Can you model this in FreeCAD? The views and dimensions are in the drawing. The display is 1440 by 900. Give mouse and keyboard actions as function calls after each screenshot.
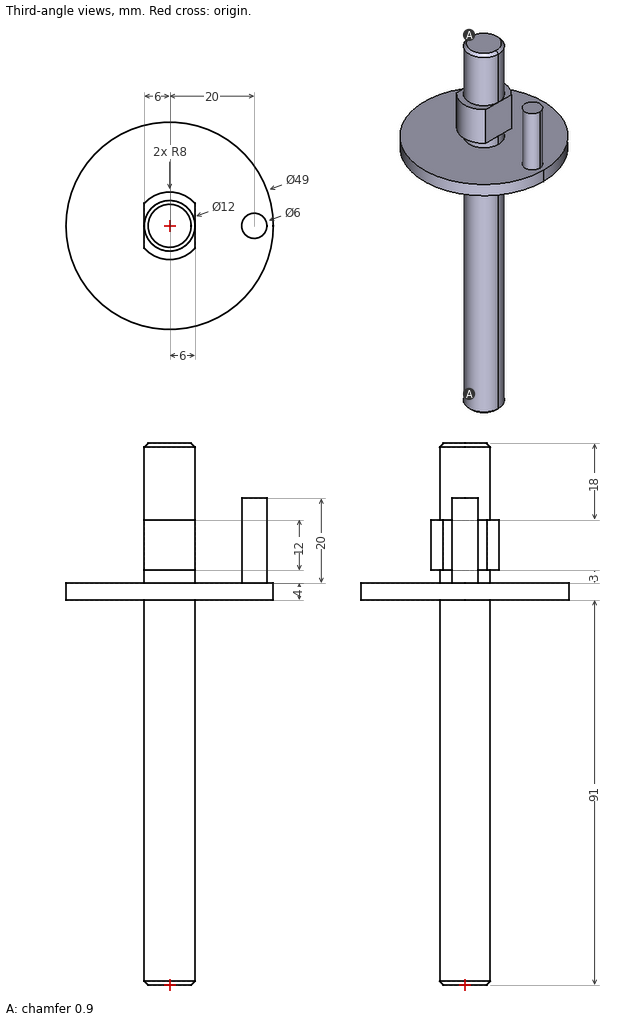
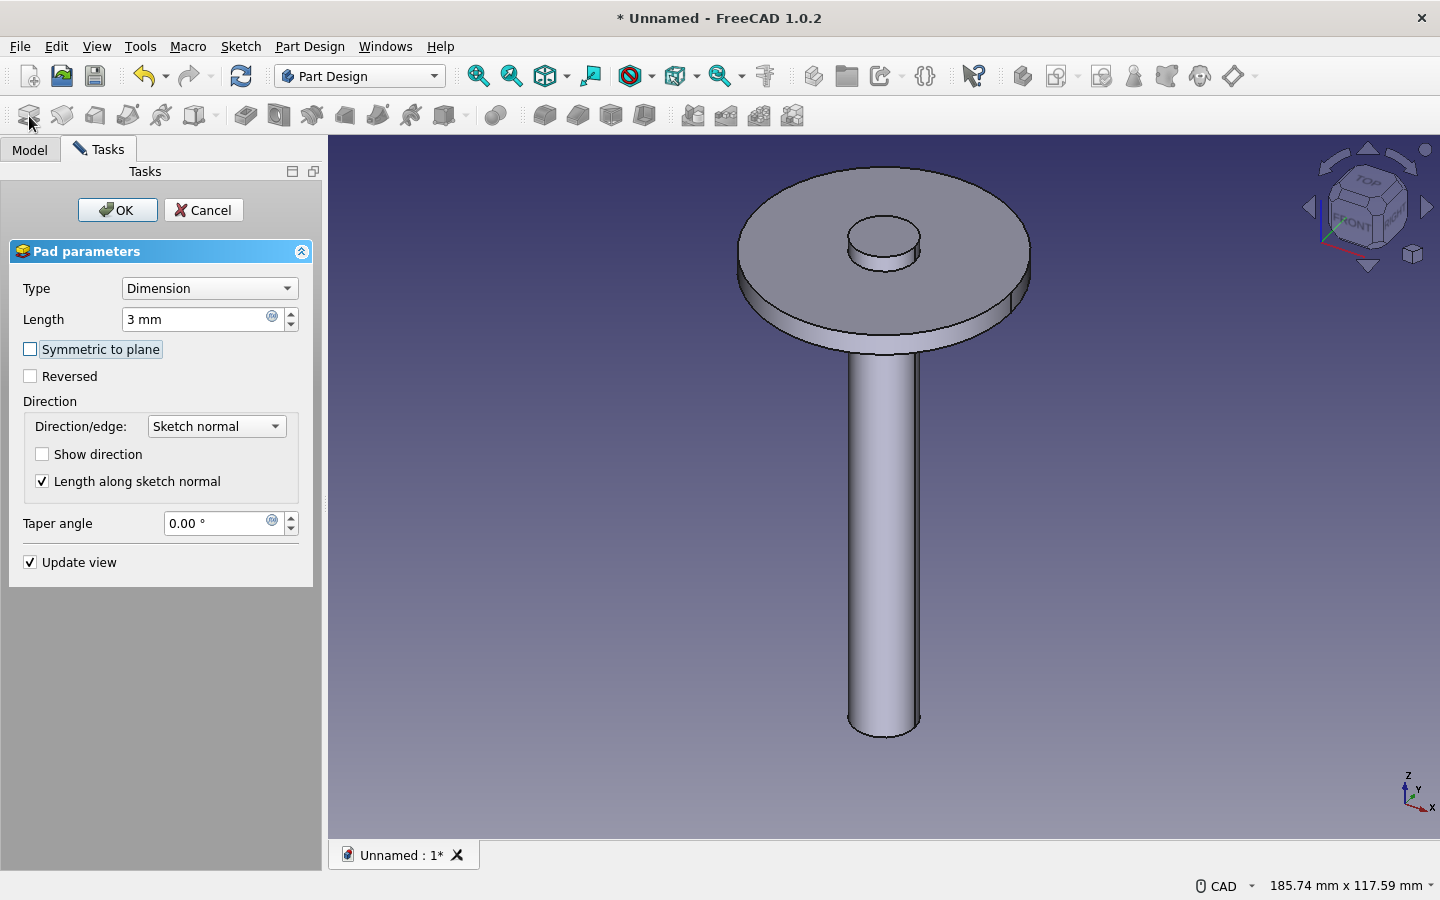
click(118, 210)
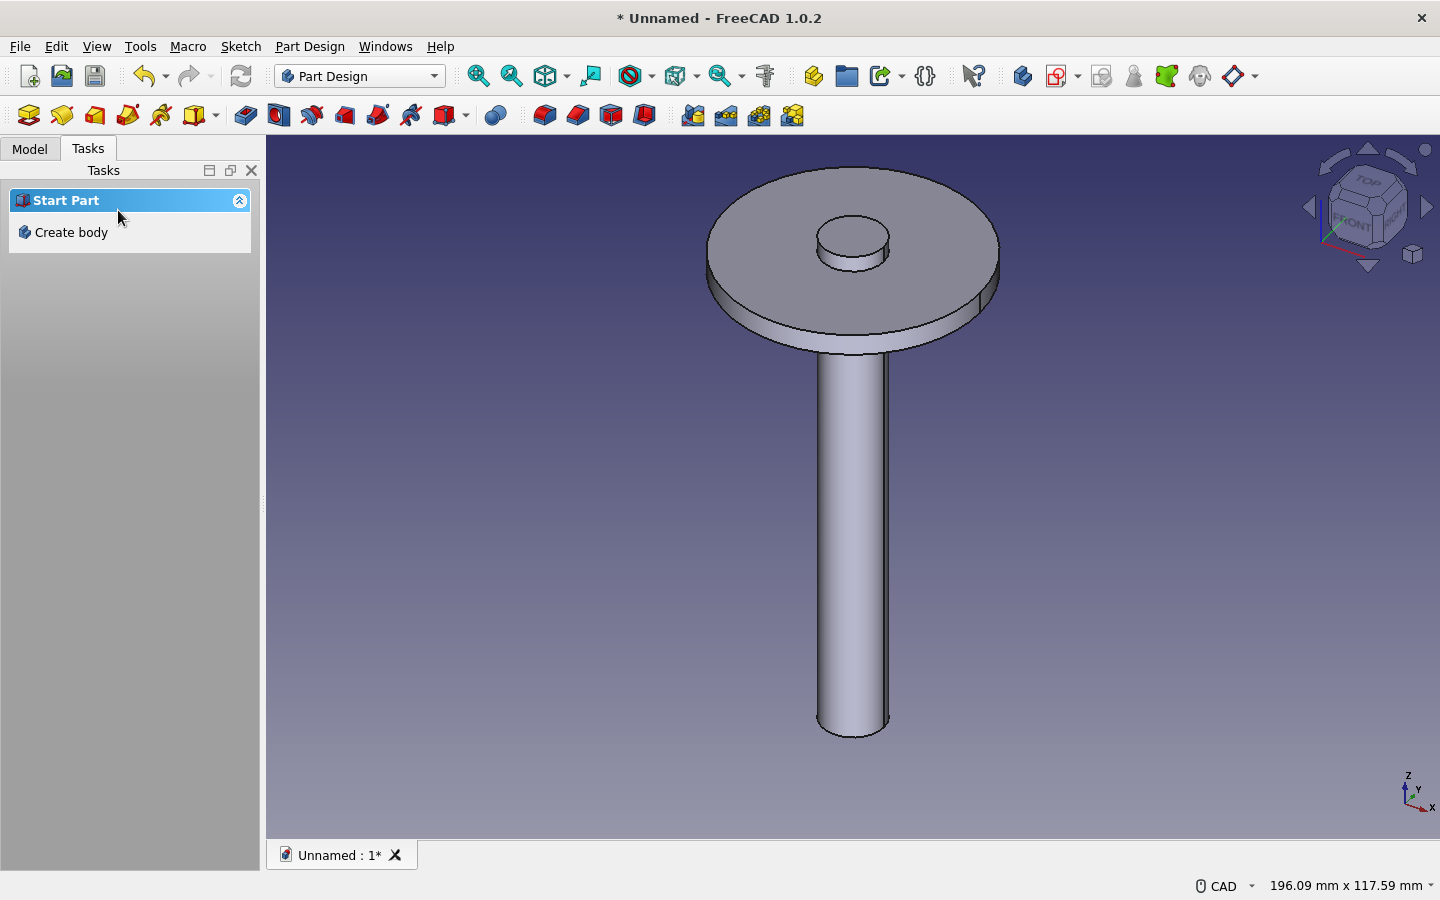
key(v)
key(f)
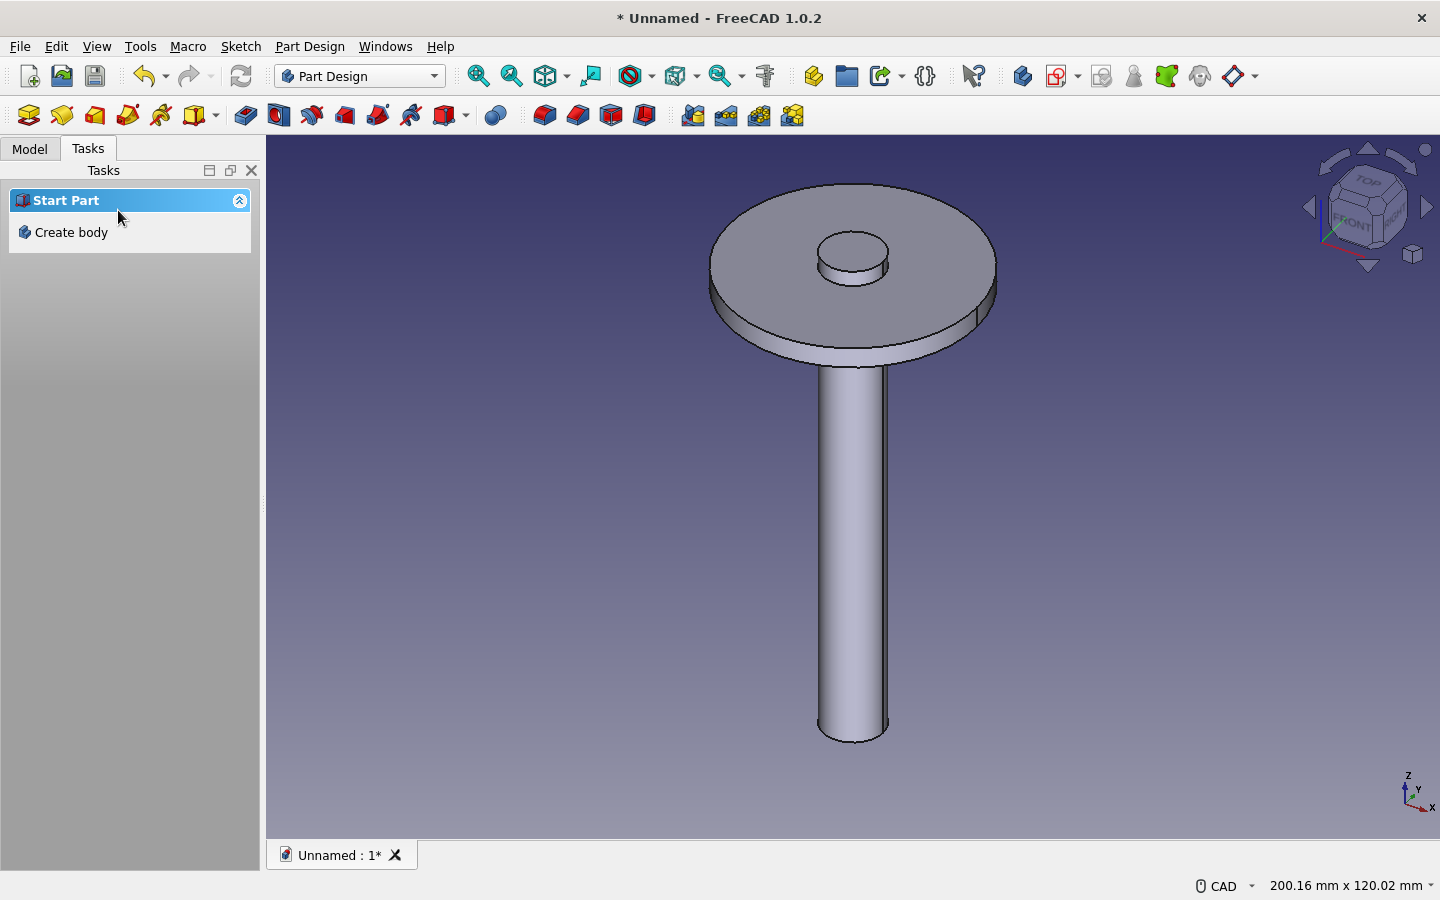
click(853, 251)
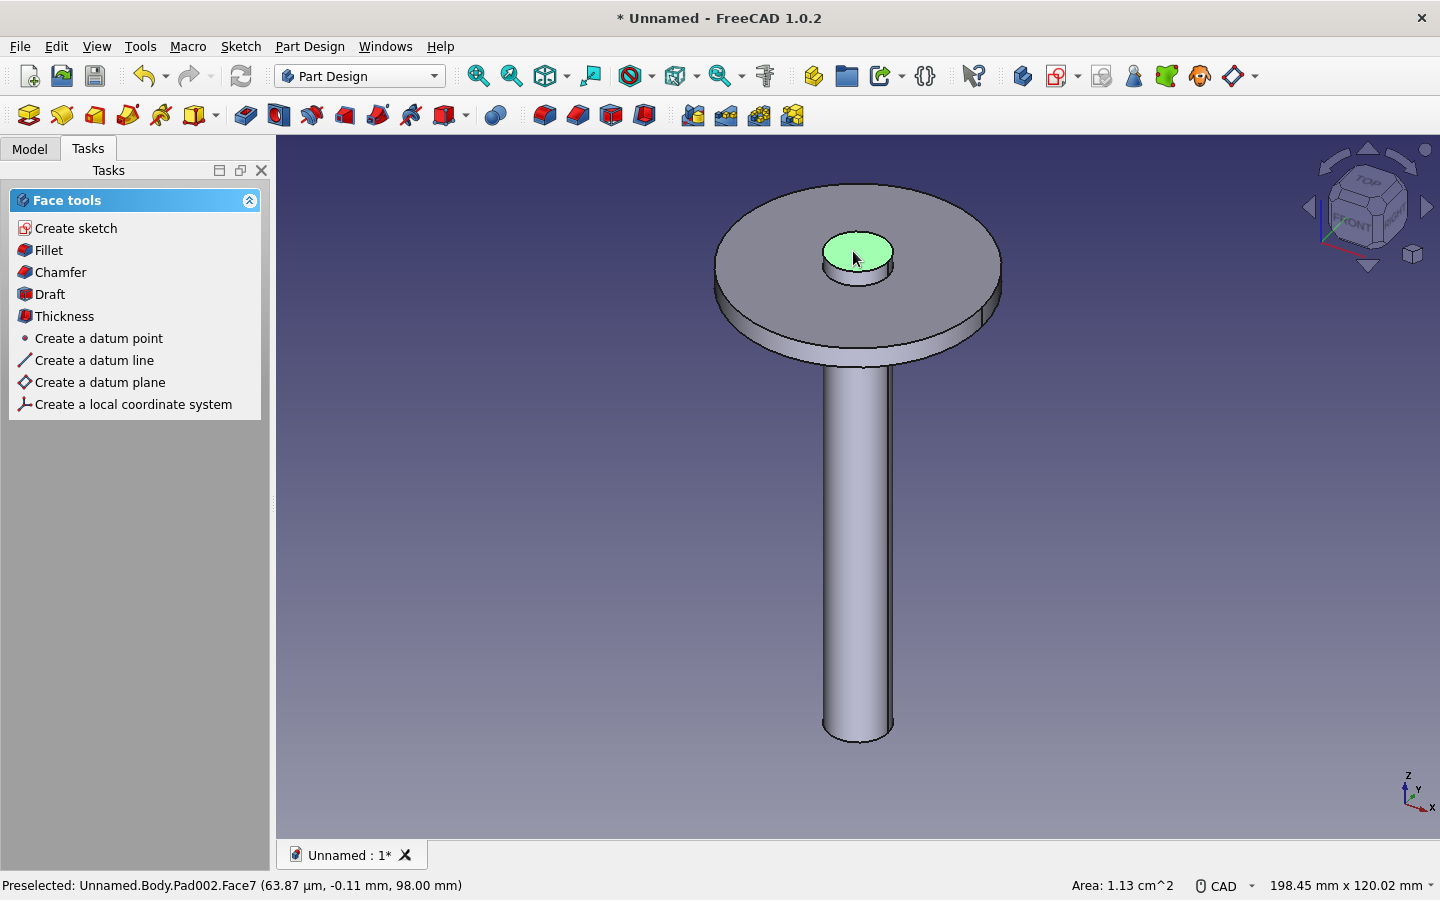
click(1056, 76)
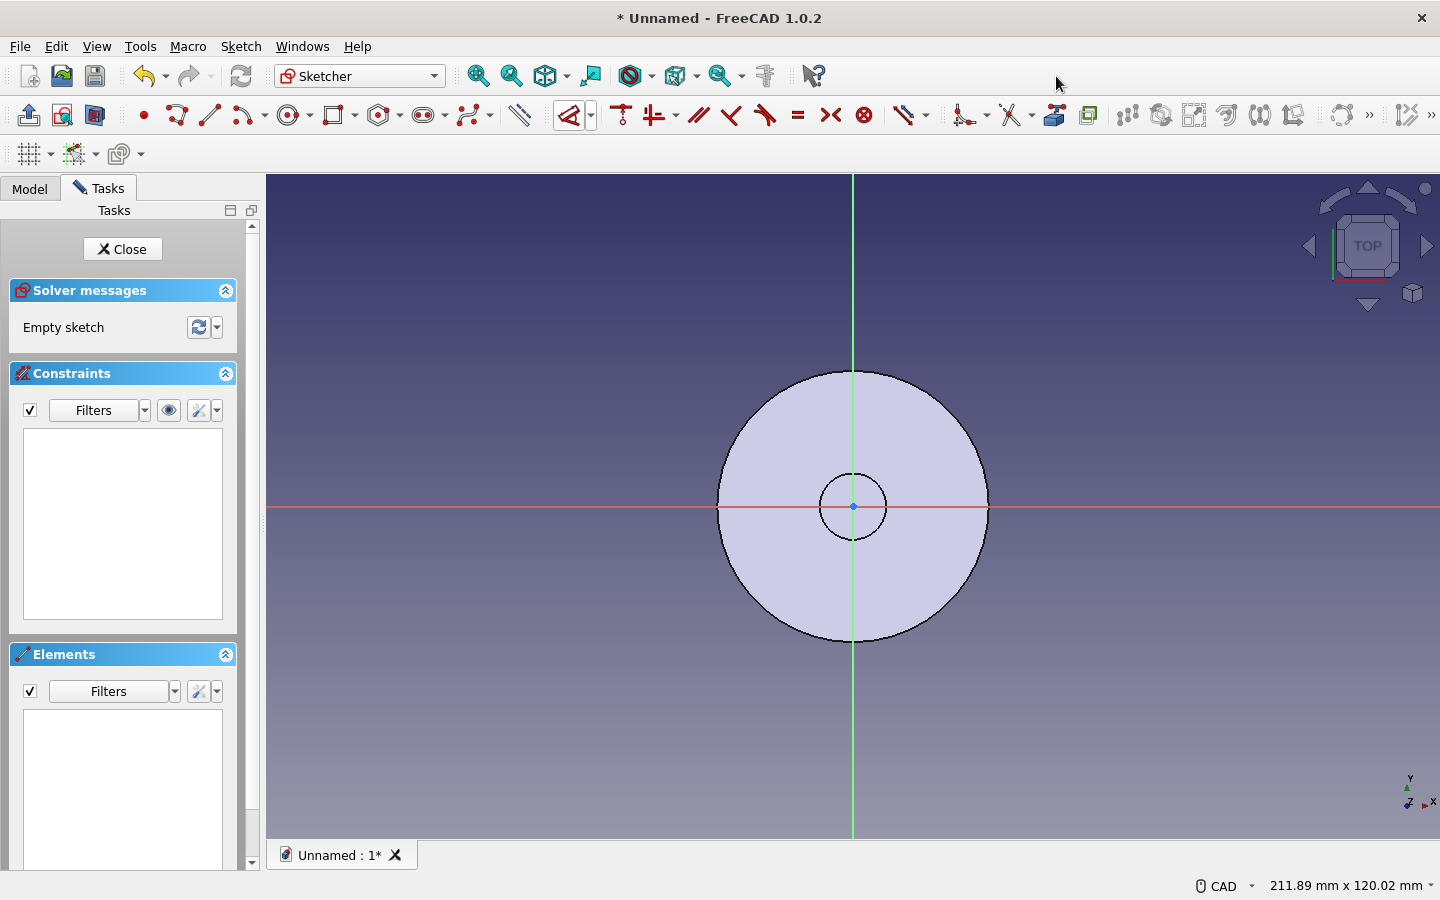
scroll(870, 506, up, 8)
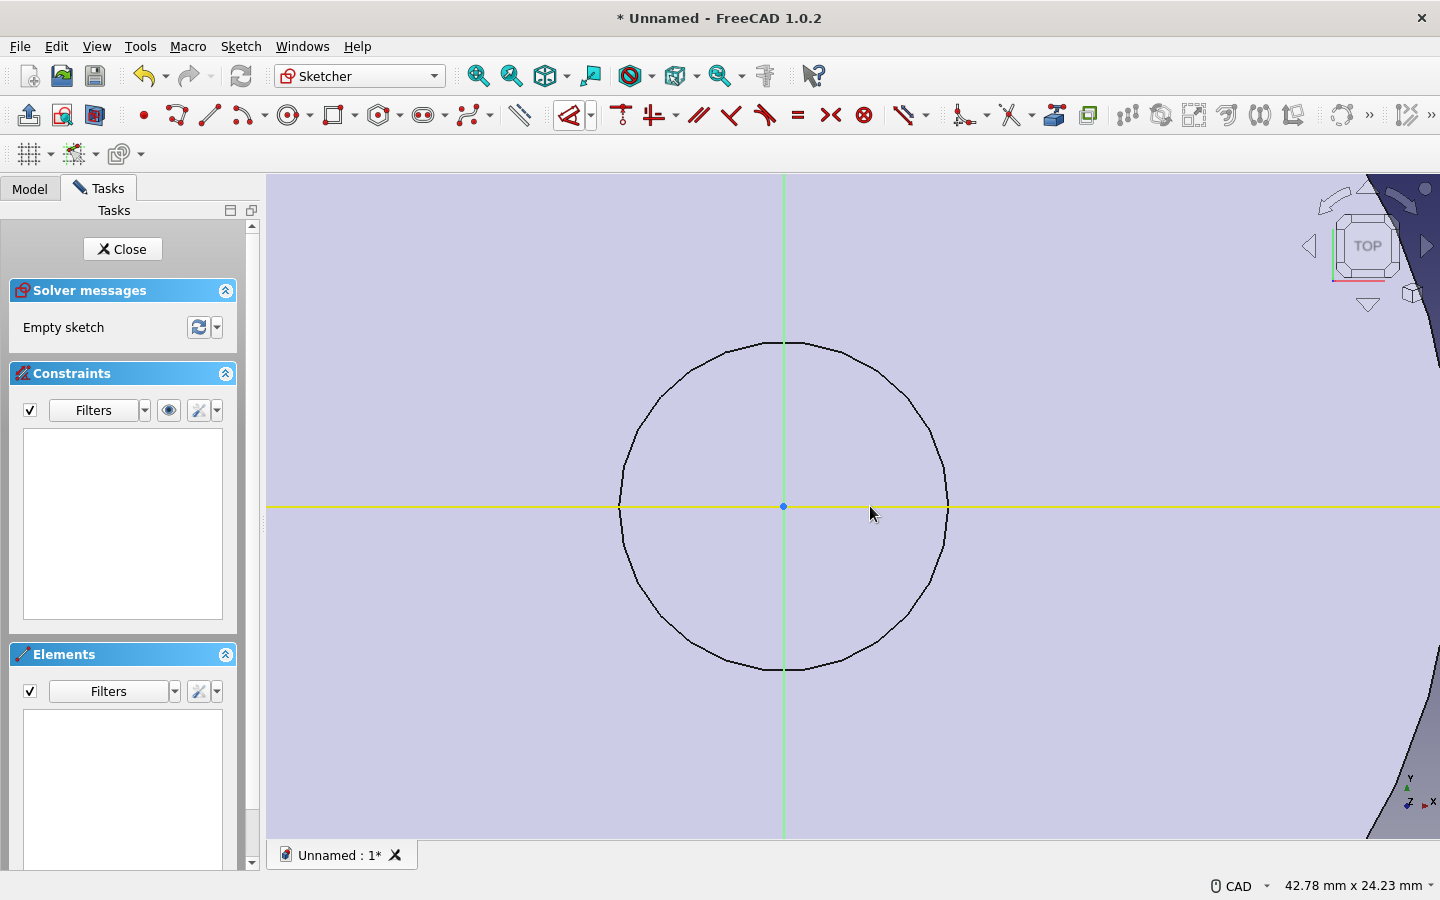
key(g)
key(l)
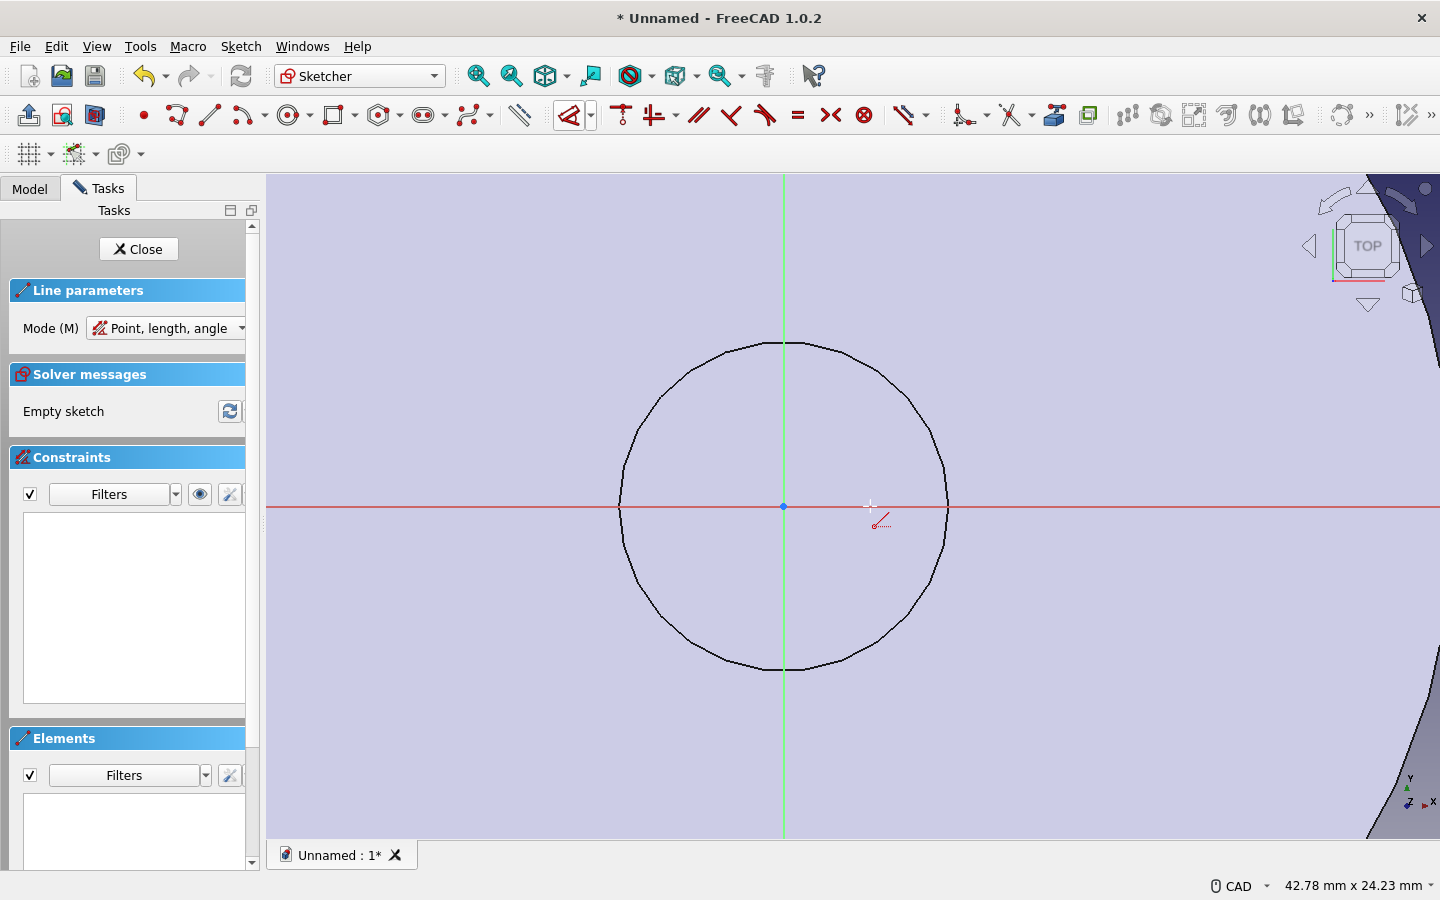
click(948, 652)
click(948, 361)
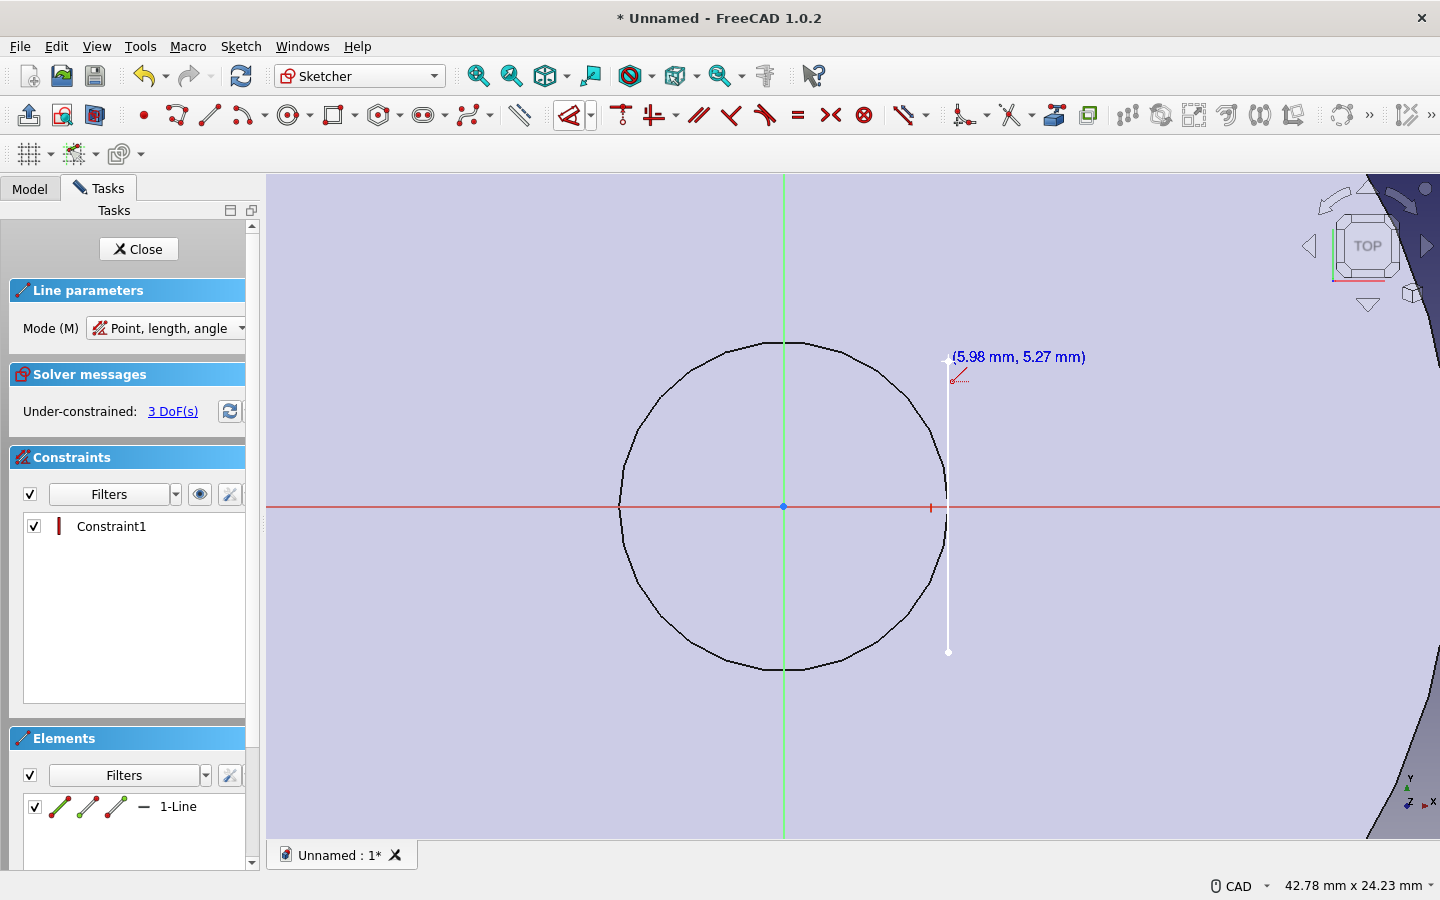
click(619, 361)
click(619, 652)